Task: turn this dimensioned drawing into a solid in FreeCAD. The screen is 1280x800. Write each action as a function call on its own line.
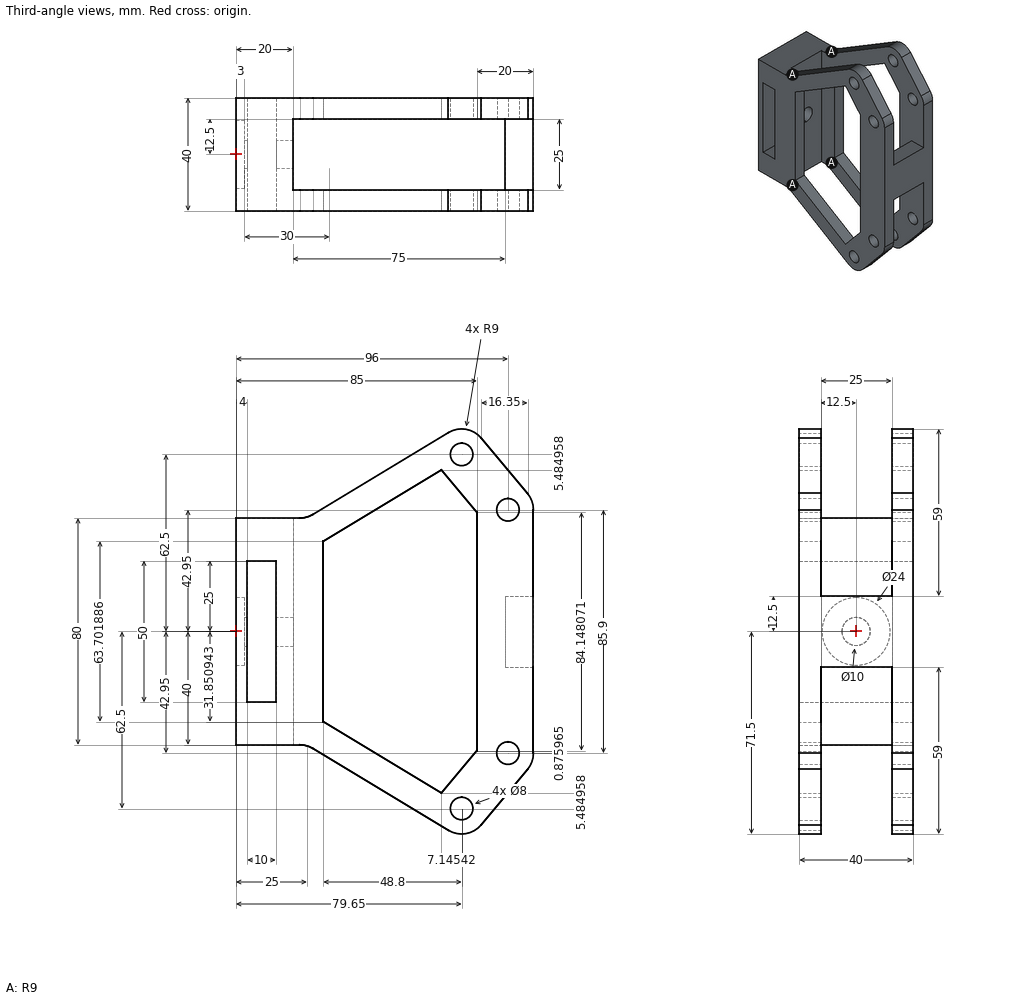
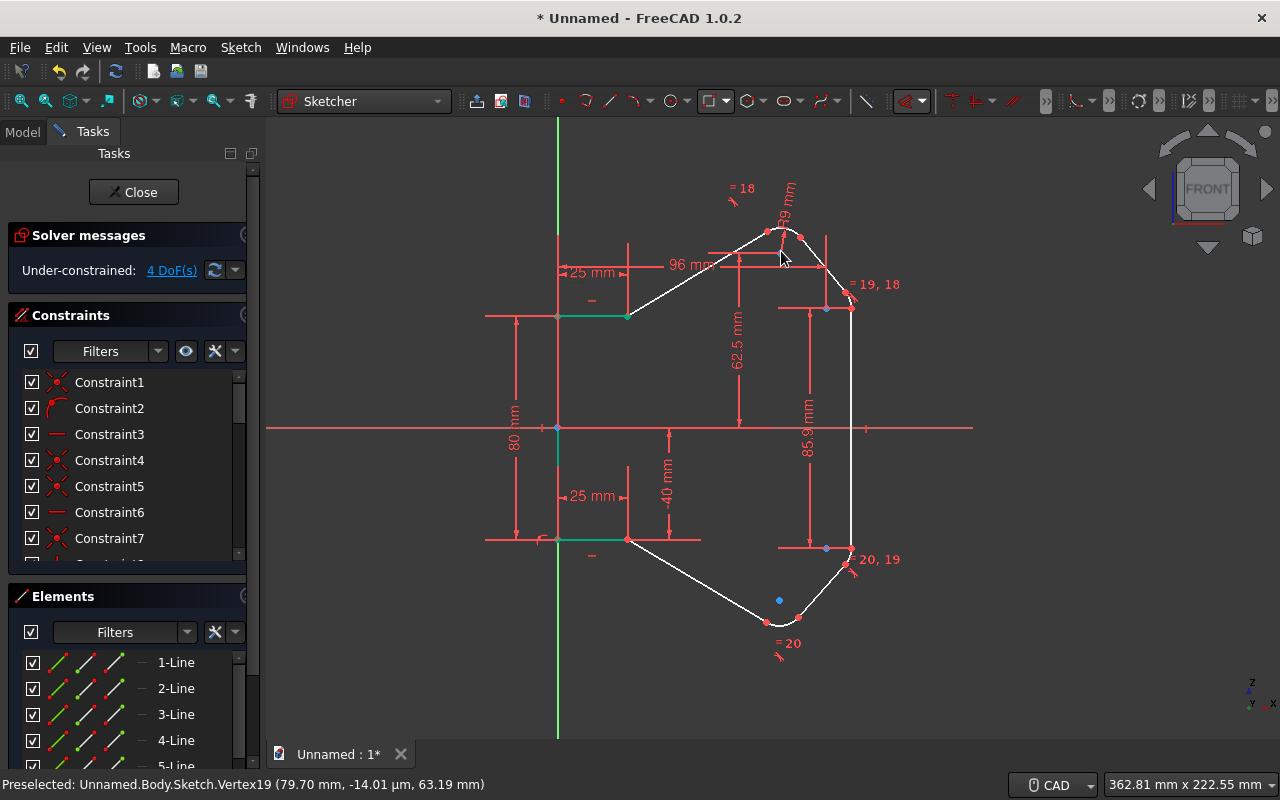
click(780, 601)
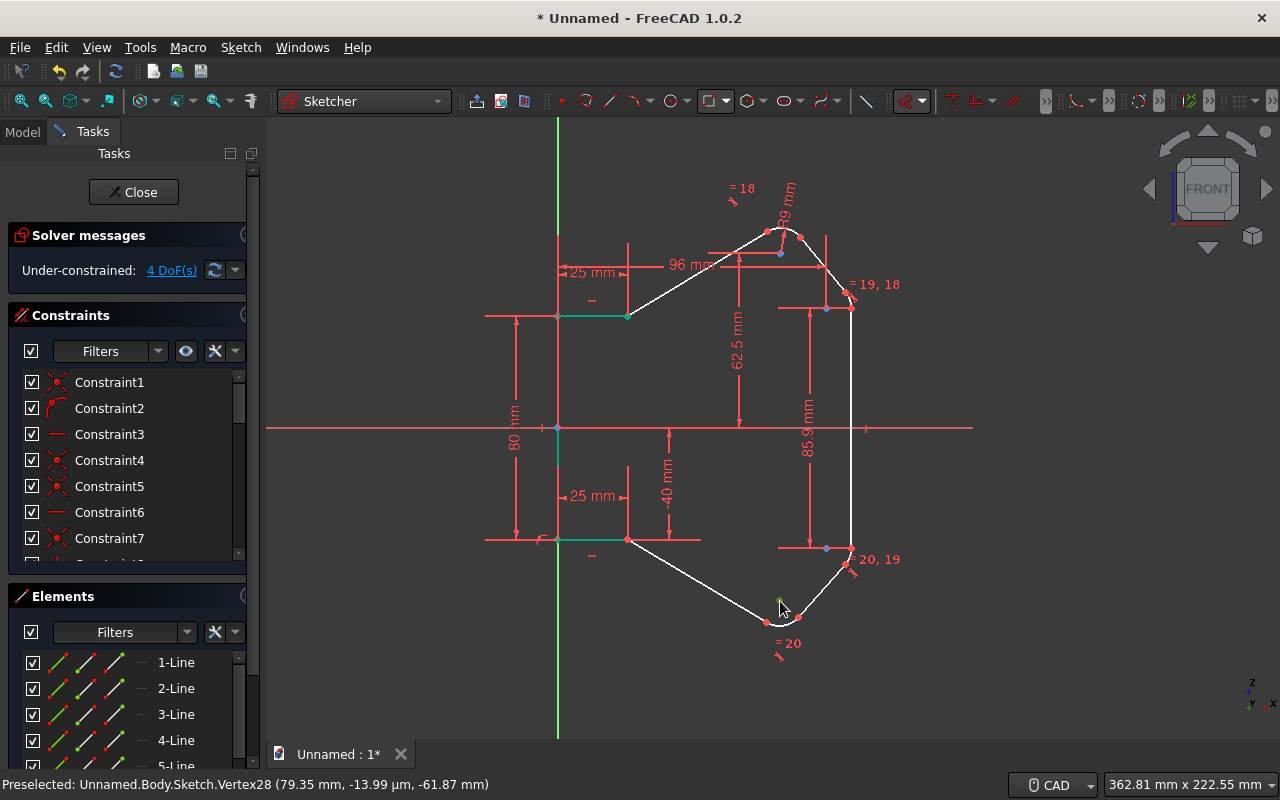
key(i)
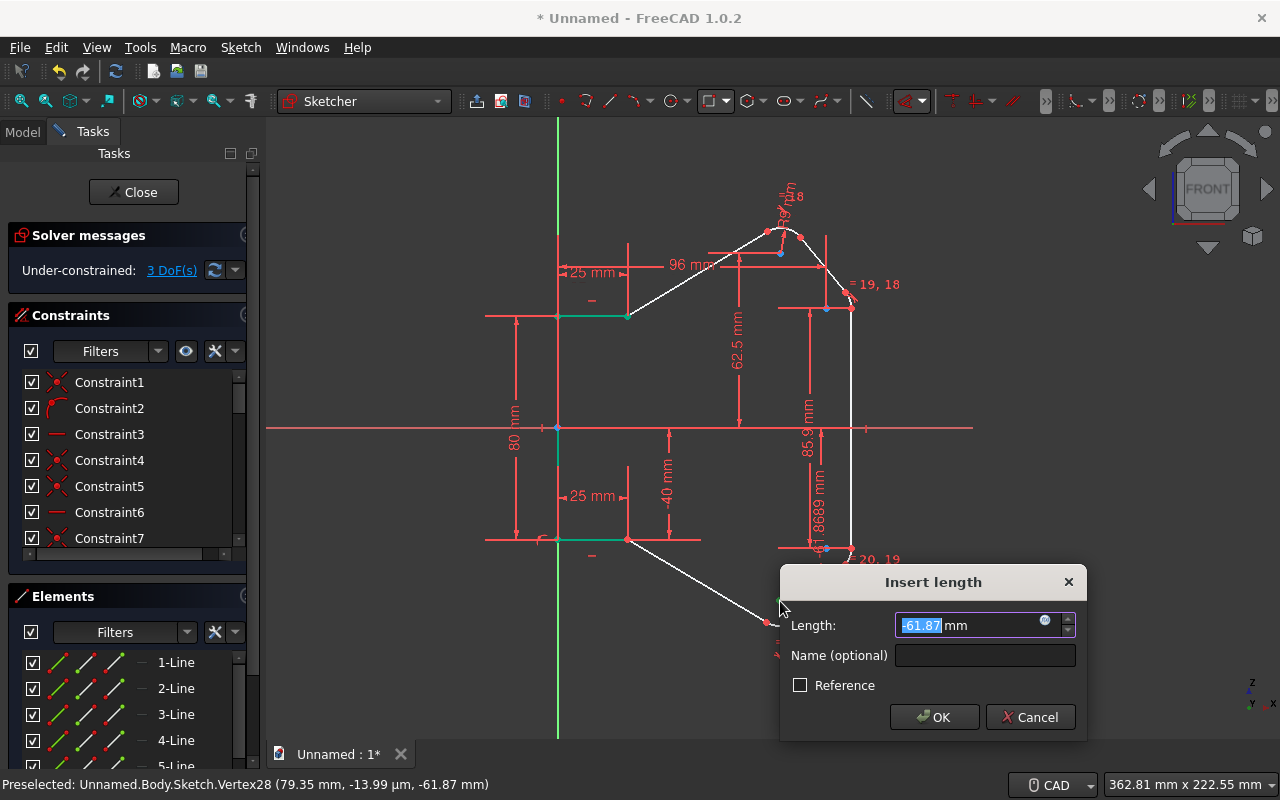
text(-62.5)
key(Return)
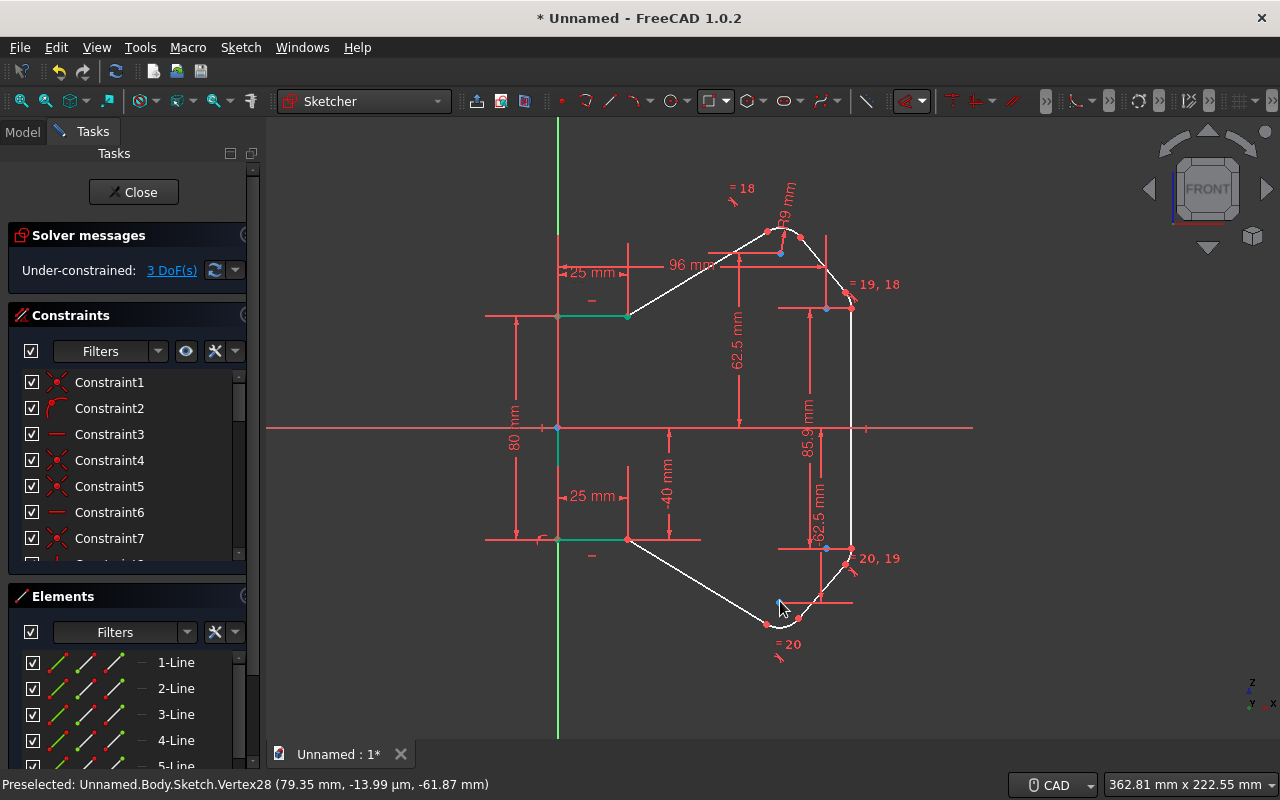
click(851, 308)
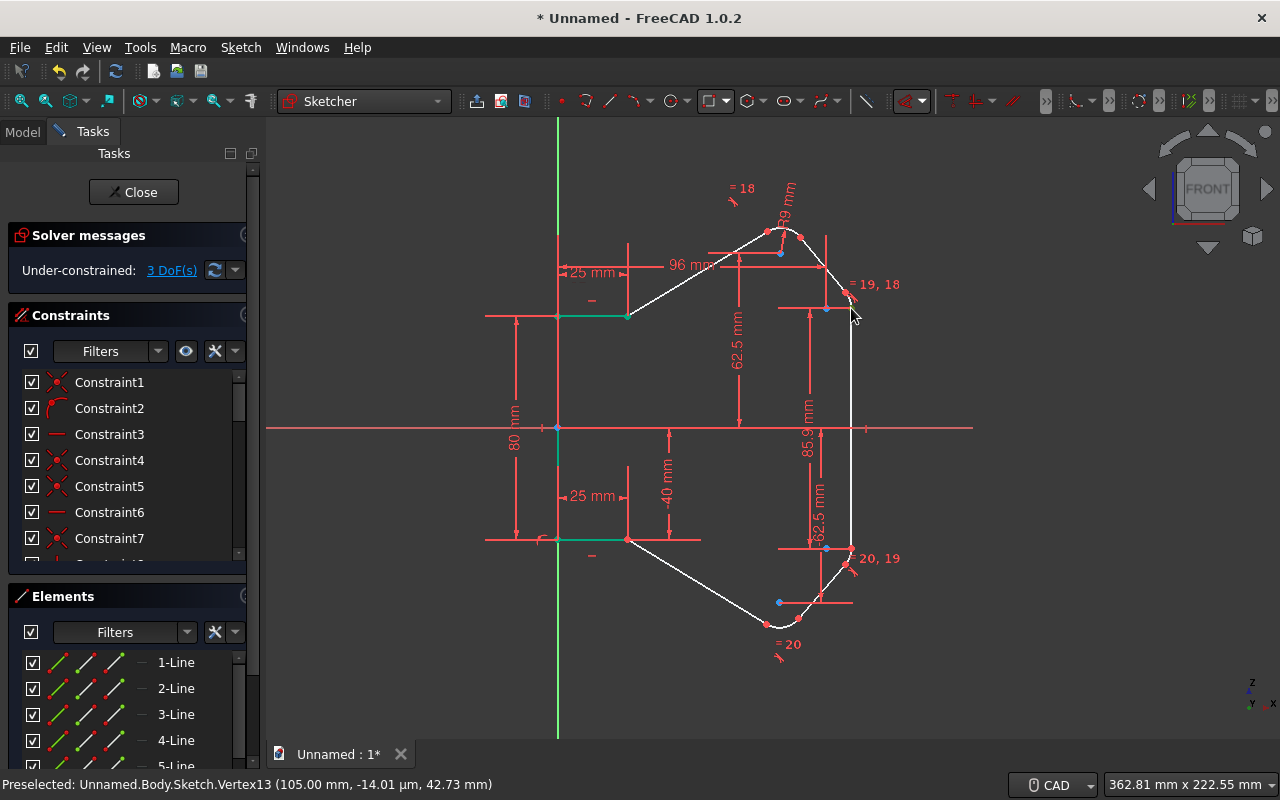
key(i)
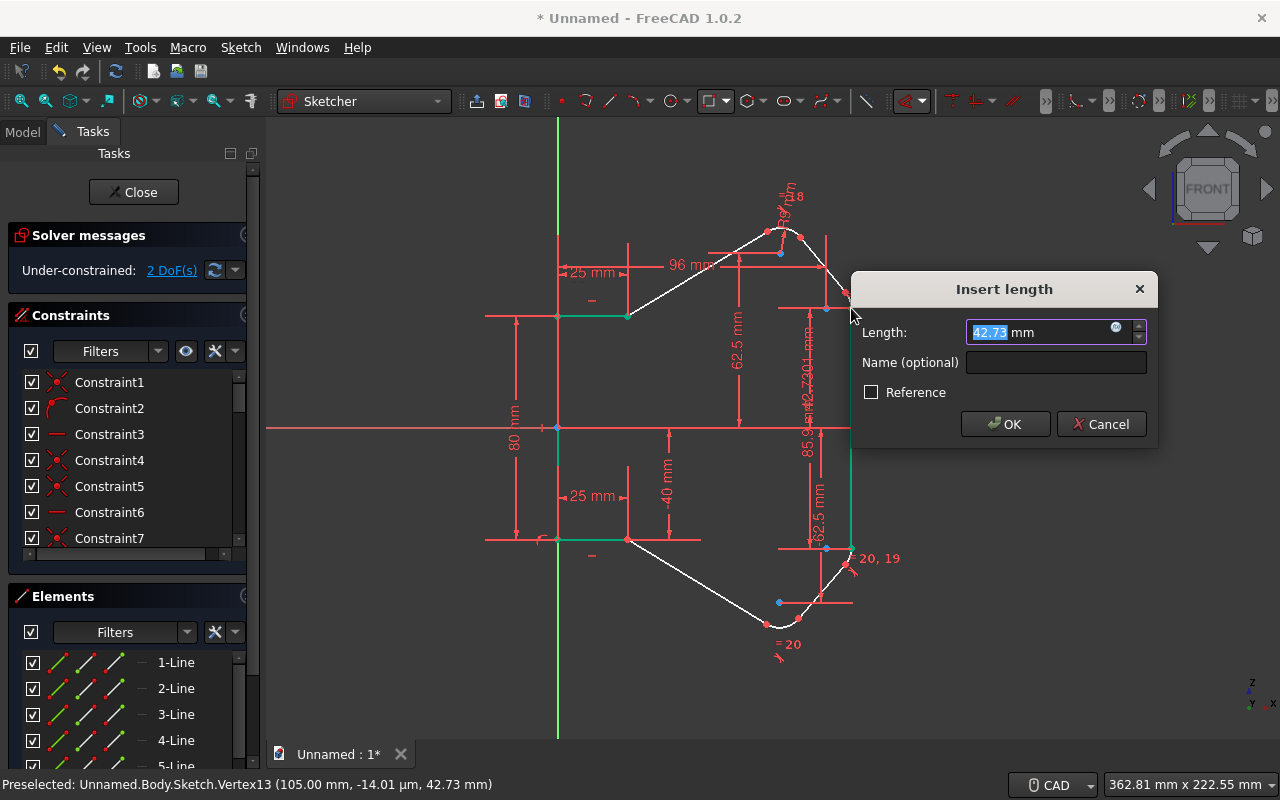
text(42.95)
key(Return)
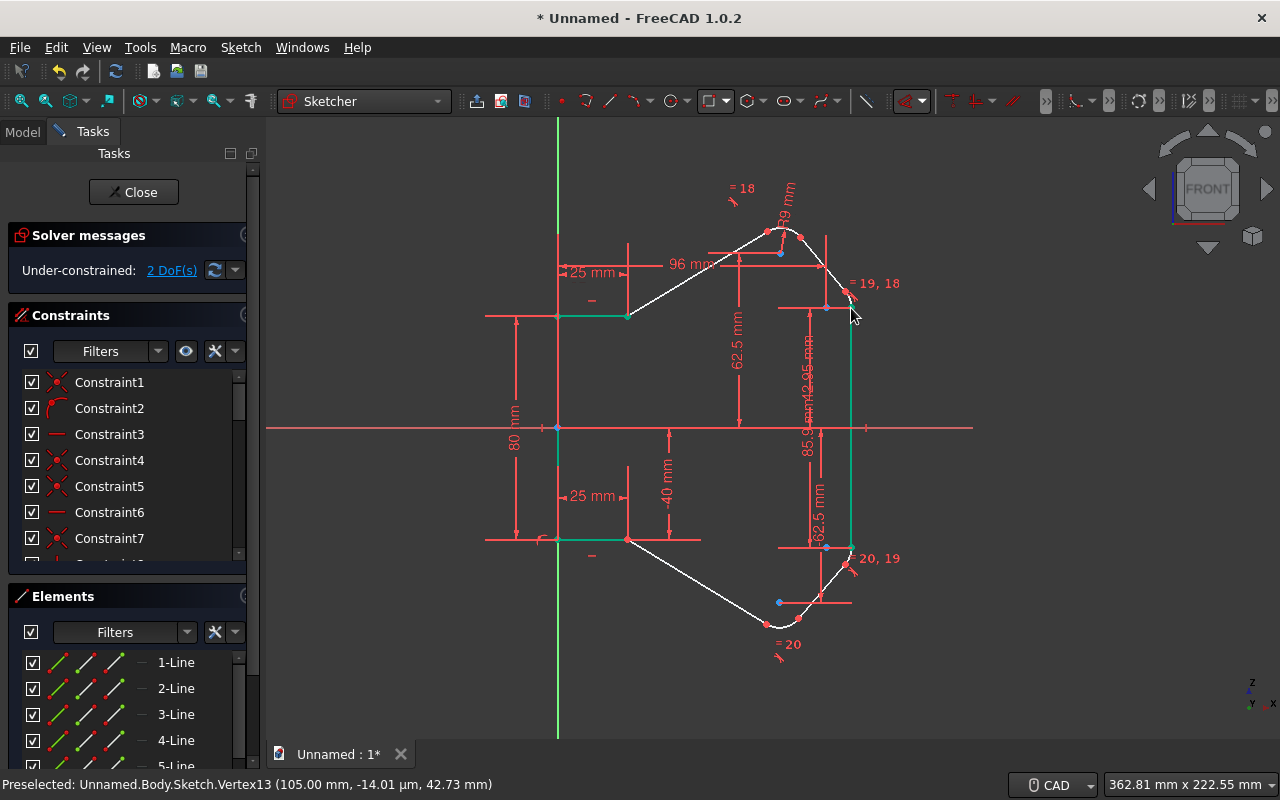
click(814, 254)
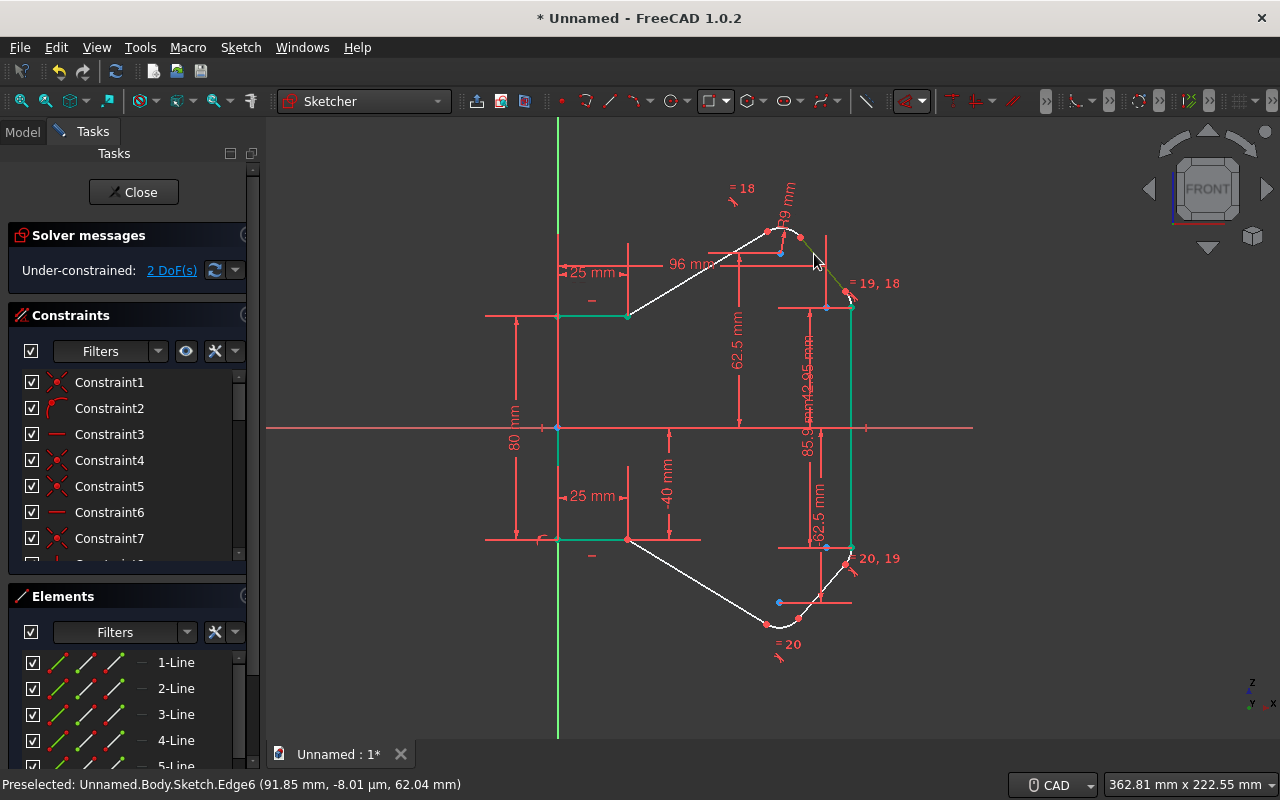
key(l)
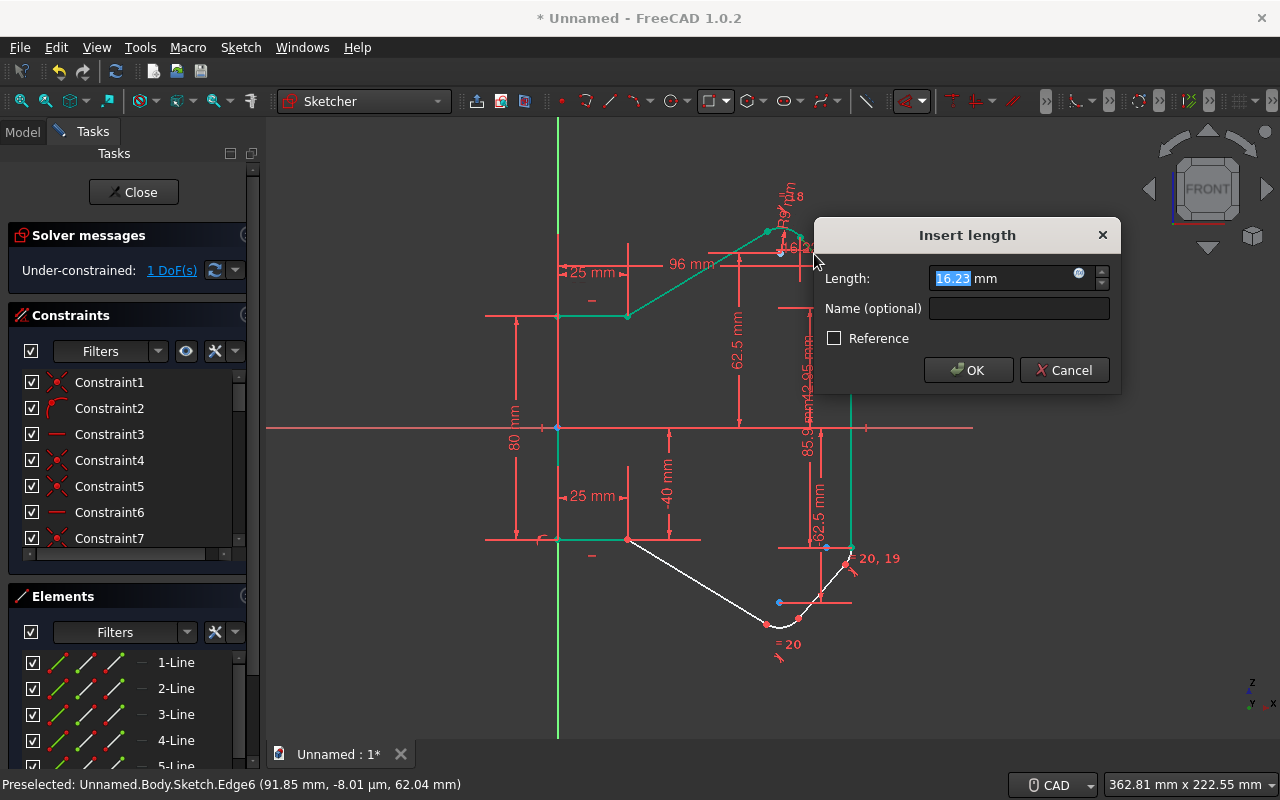
text(16.35)
key(Return)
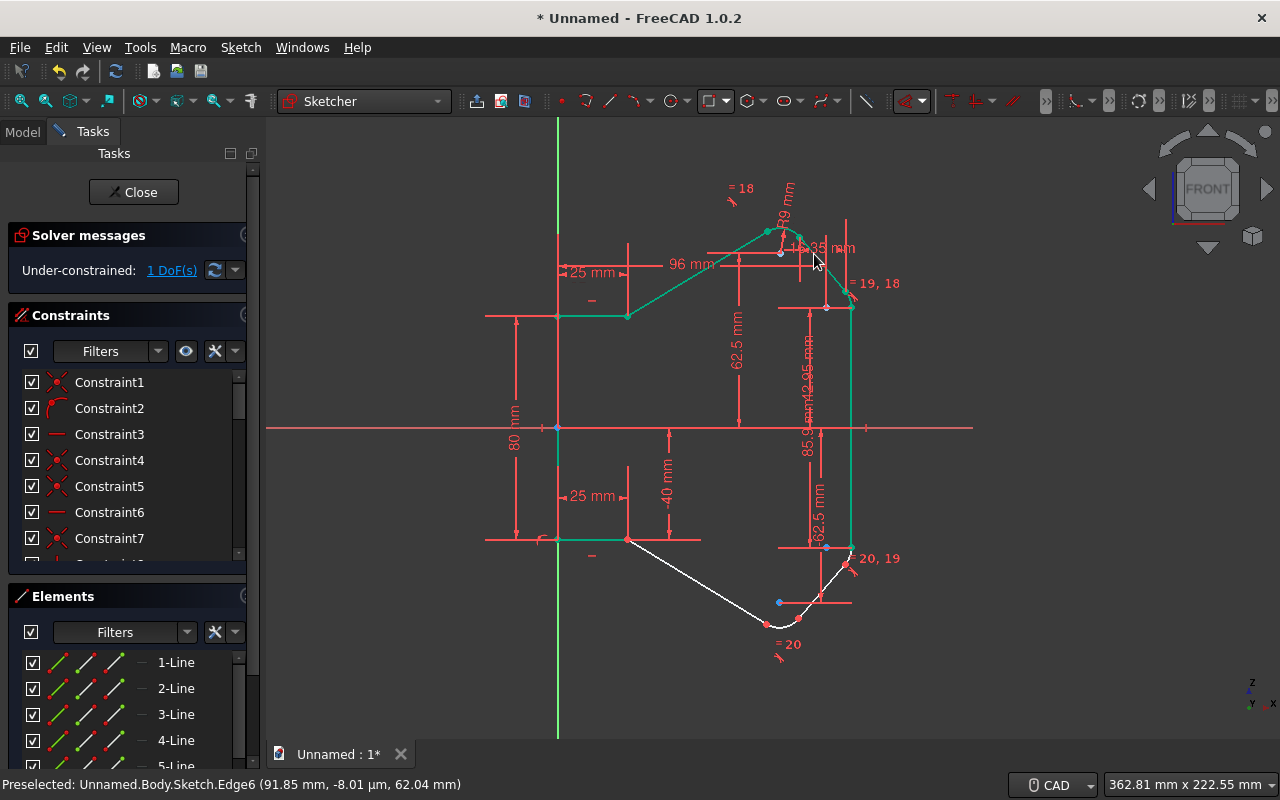
click(831, 581)